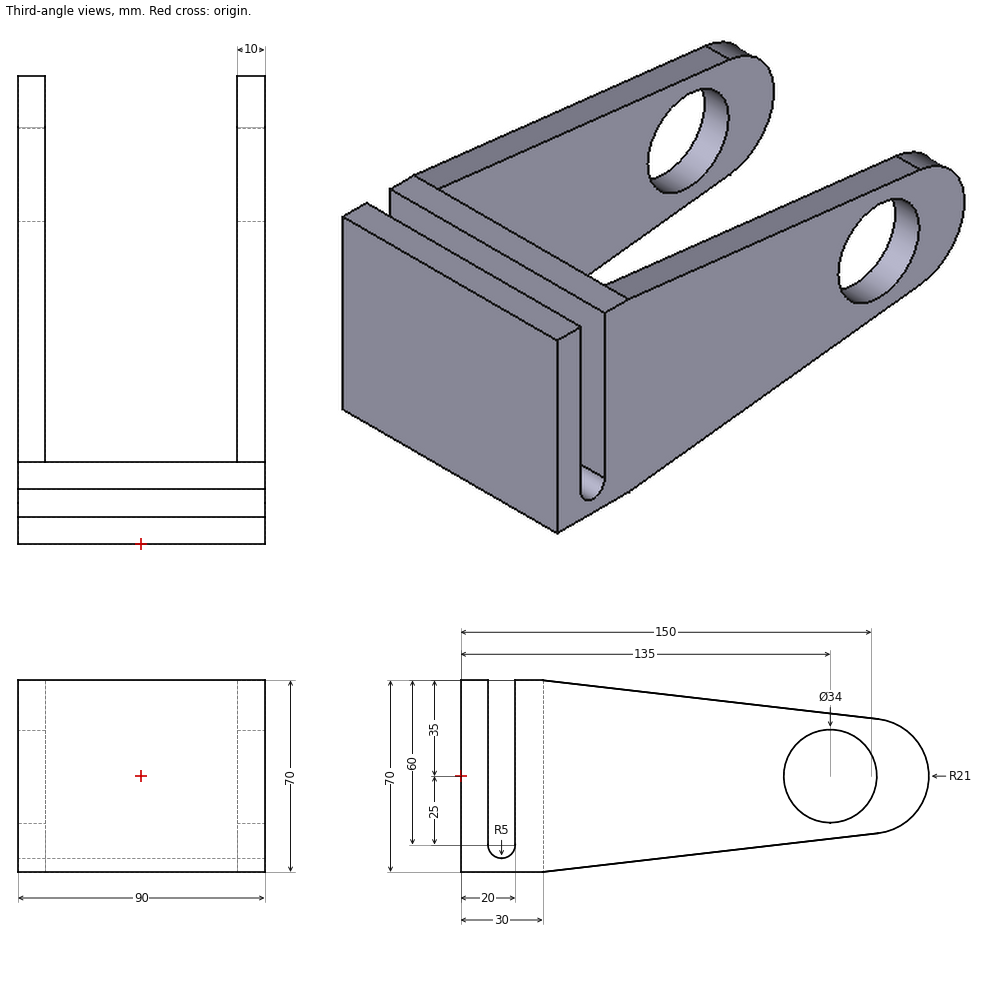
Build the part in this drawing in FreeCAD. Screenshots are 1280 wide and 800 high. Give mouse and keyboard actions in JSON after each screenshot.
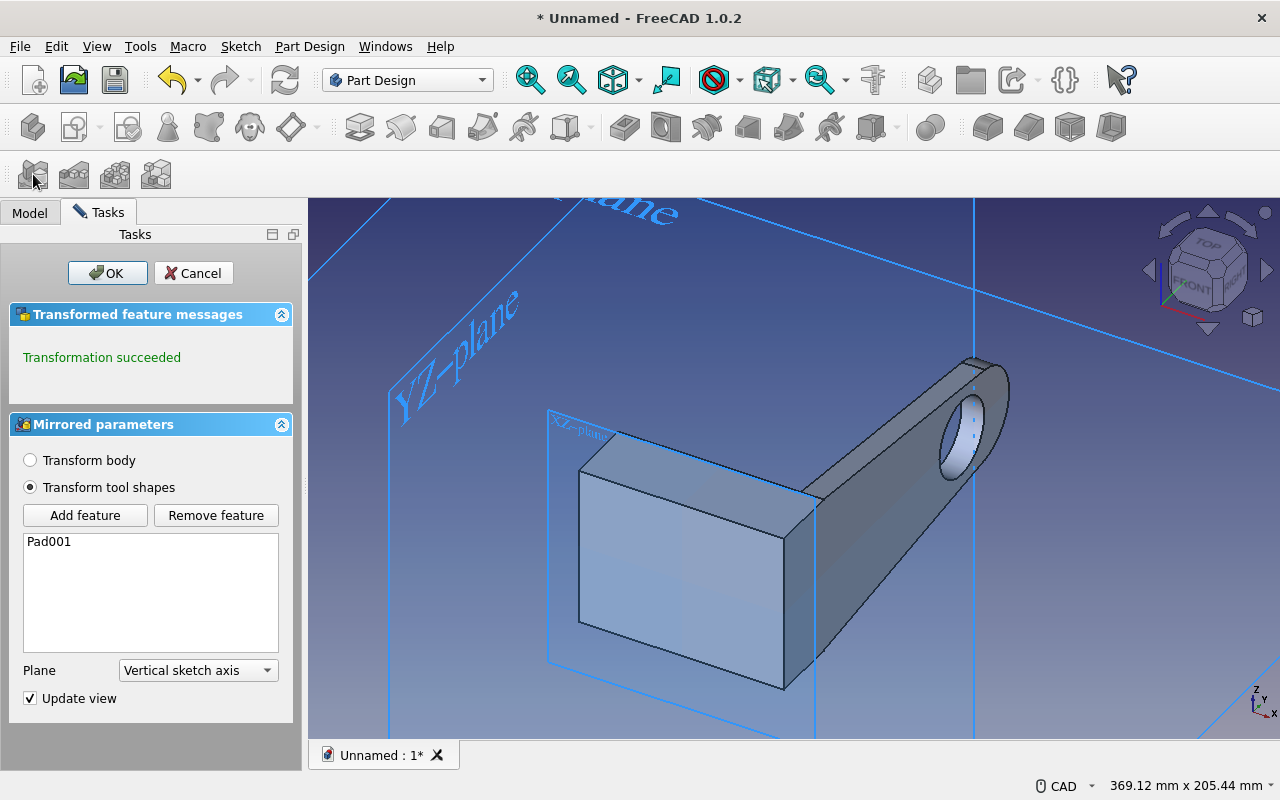
{"action": "left_click", "coordinate": [199, 670]}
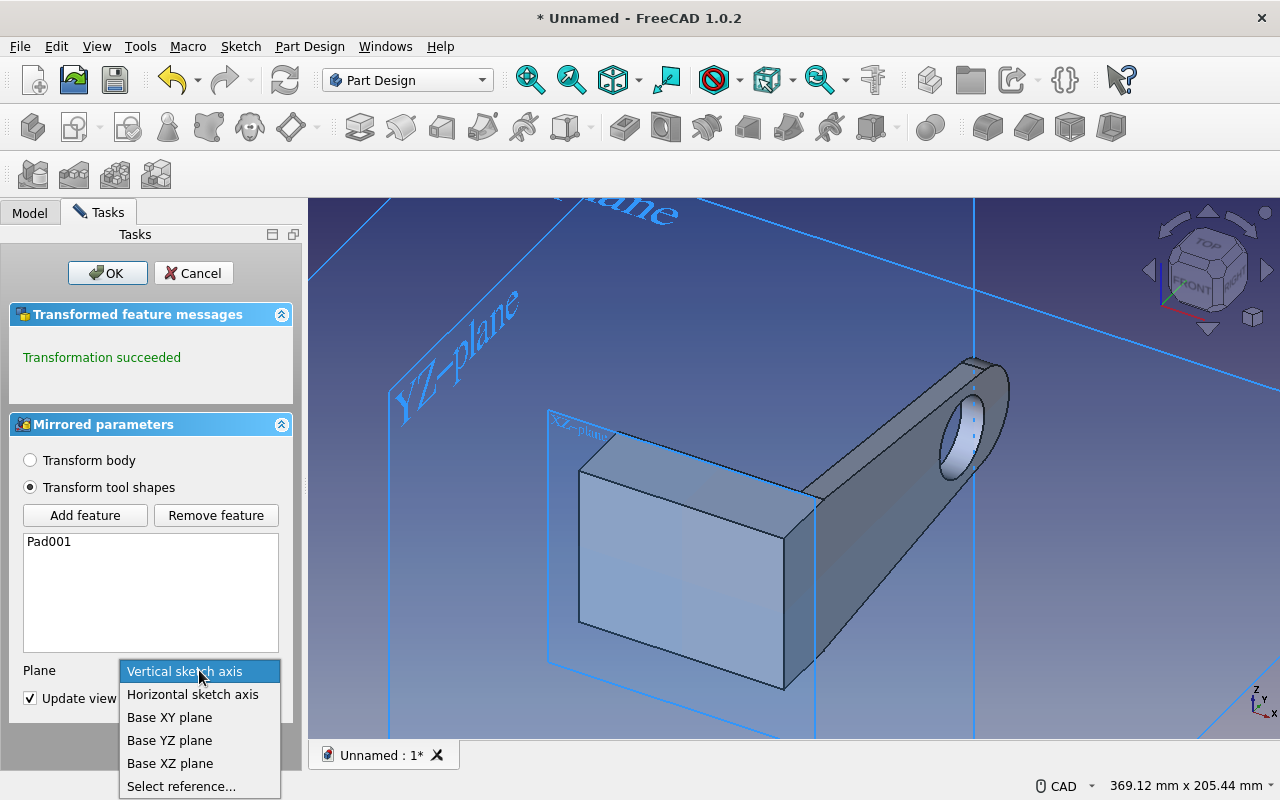
{"action": "left_click", "coordinate": [198, 740]}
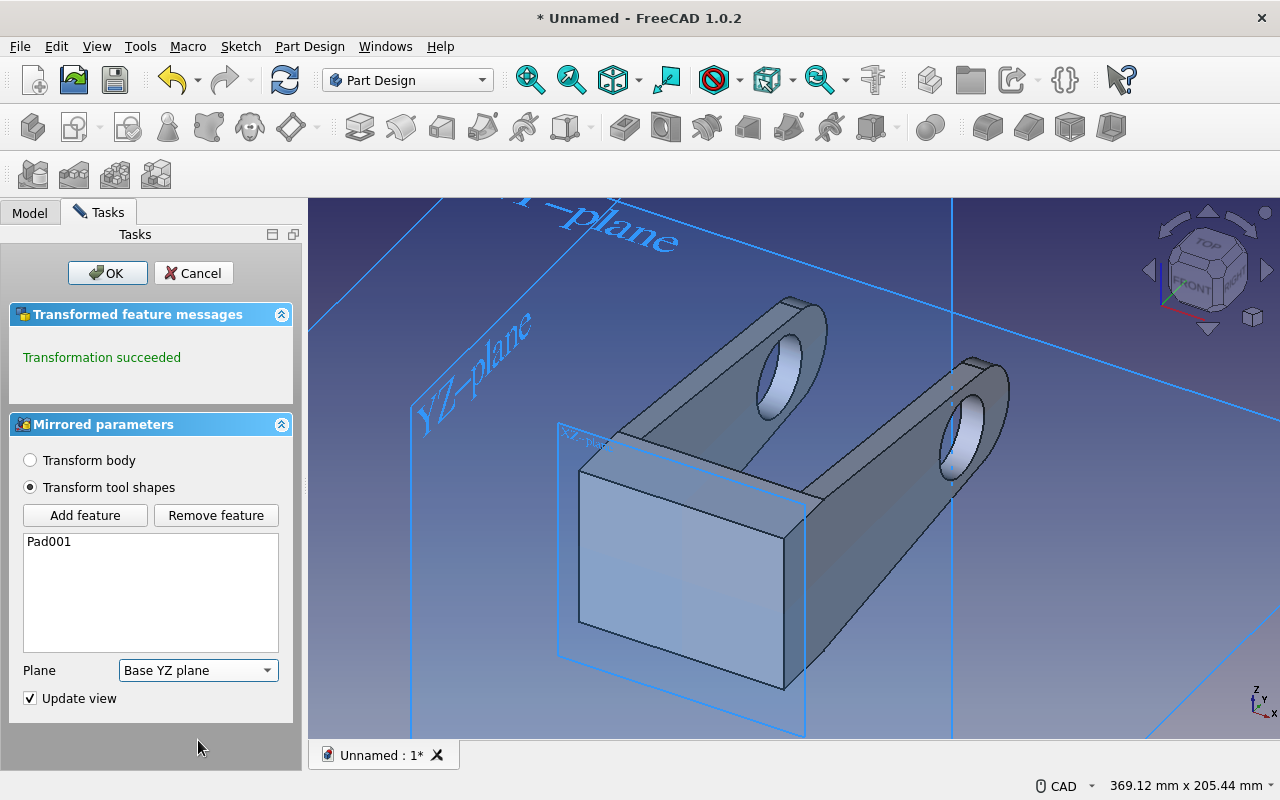
{"action": "left_click", "coordinate": [108, 273]}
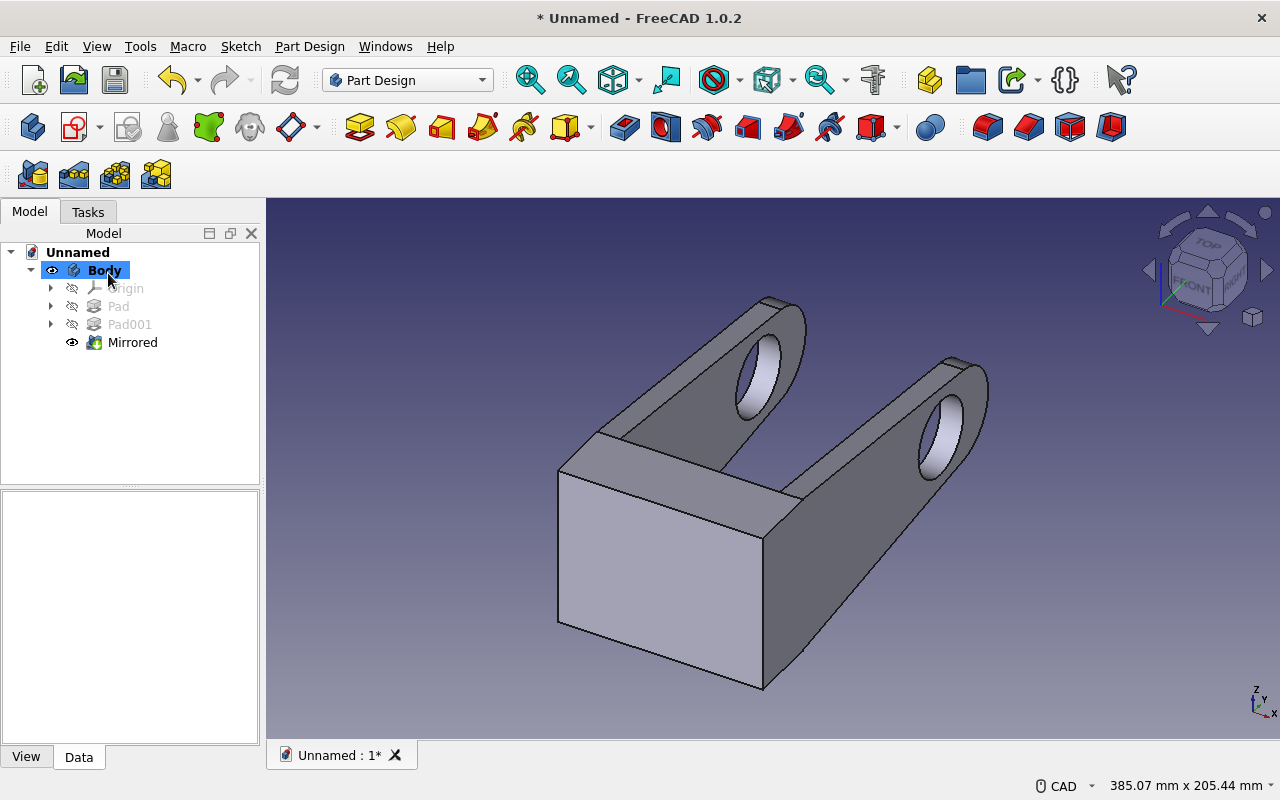
{"action": "left_click", "coordinate": [811, 565]}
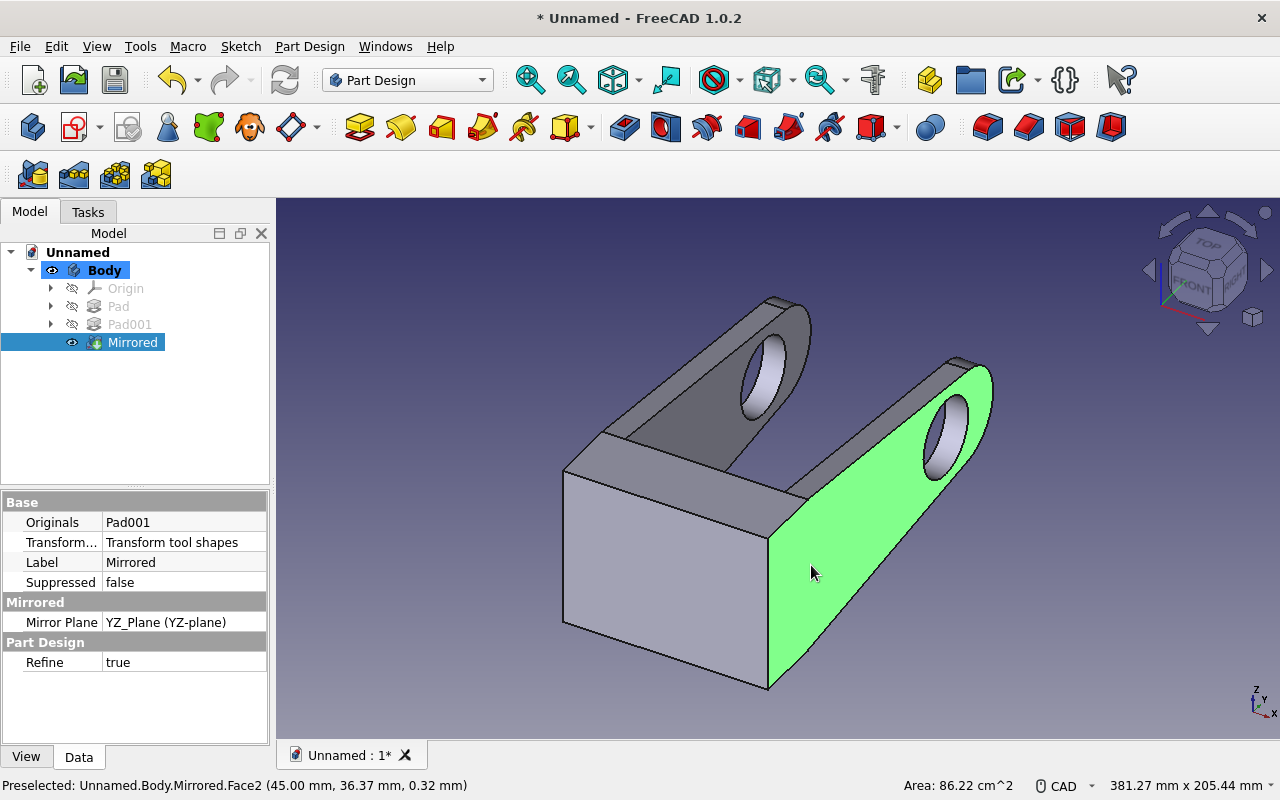
{"action": "left_click", "coordinate": [74, 128]}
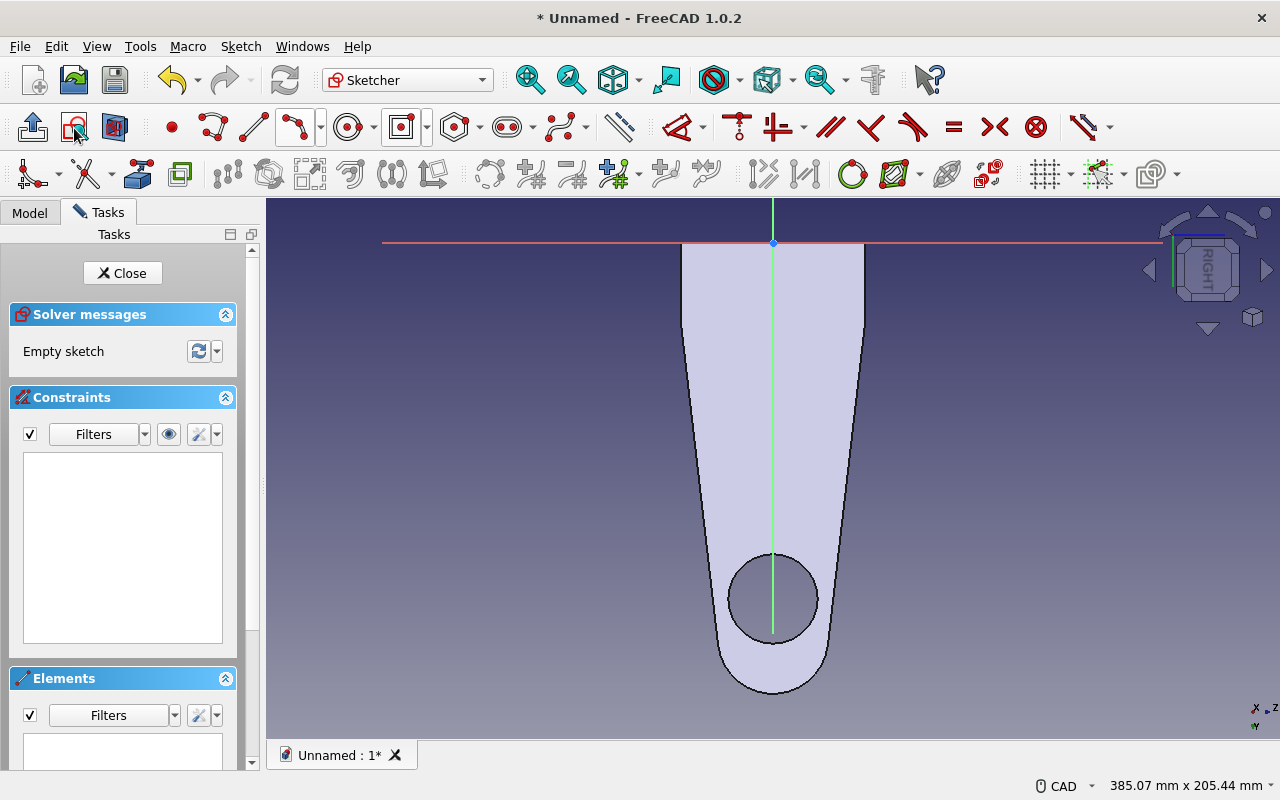
{"action": "scroll", "coordinate": [812, 226], "scroll_direction": "up", "scroll_amount": 6}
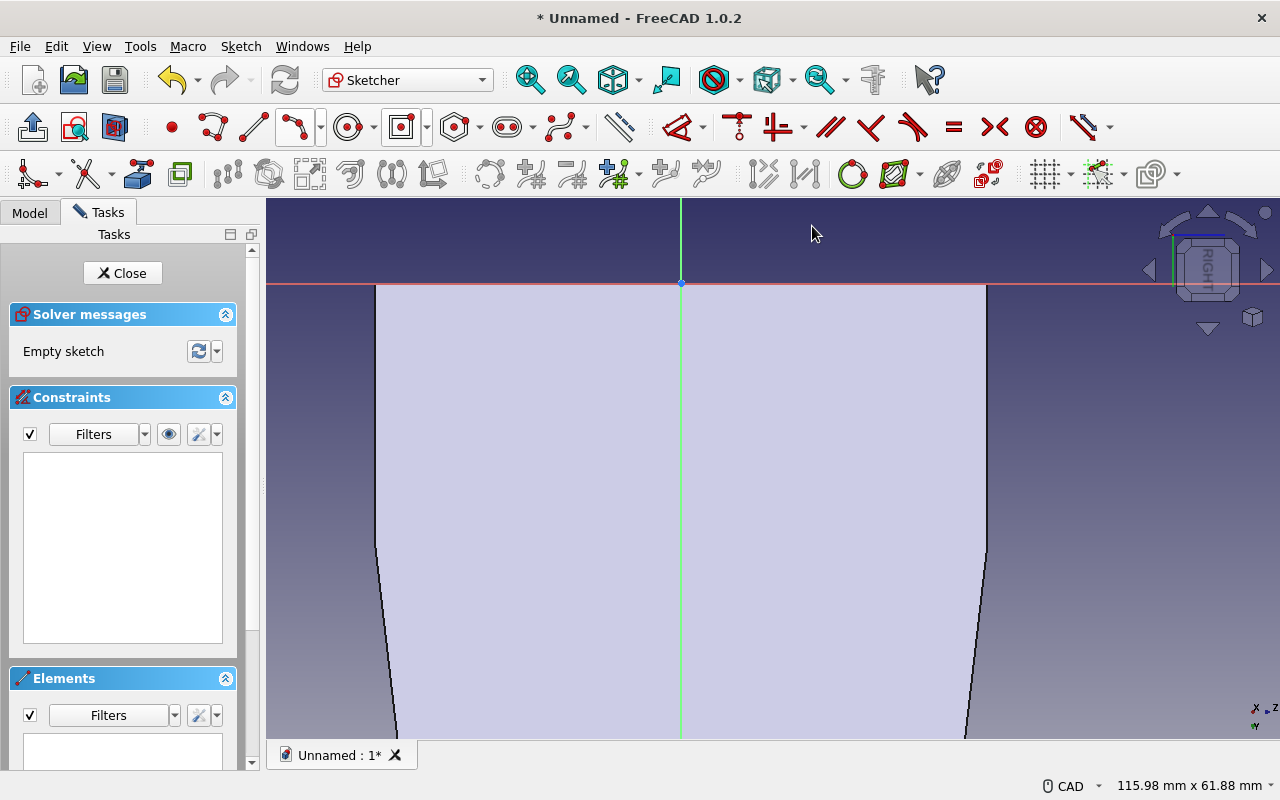
{"action": "left_click", "coordinate": [213, 128]}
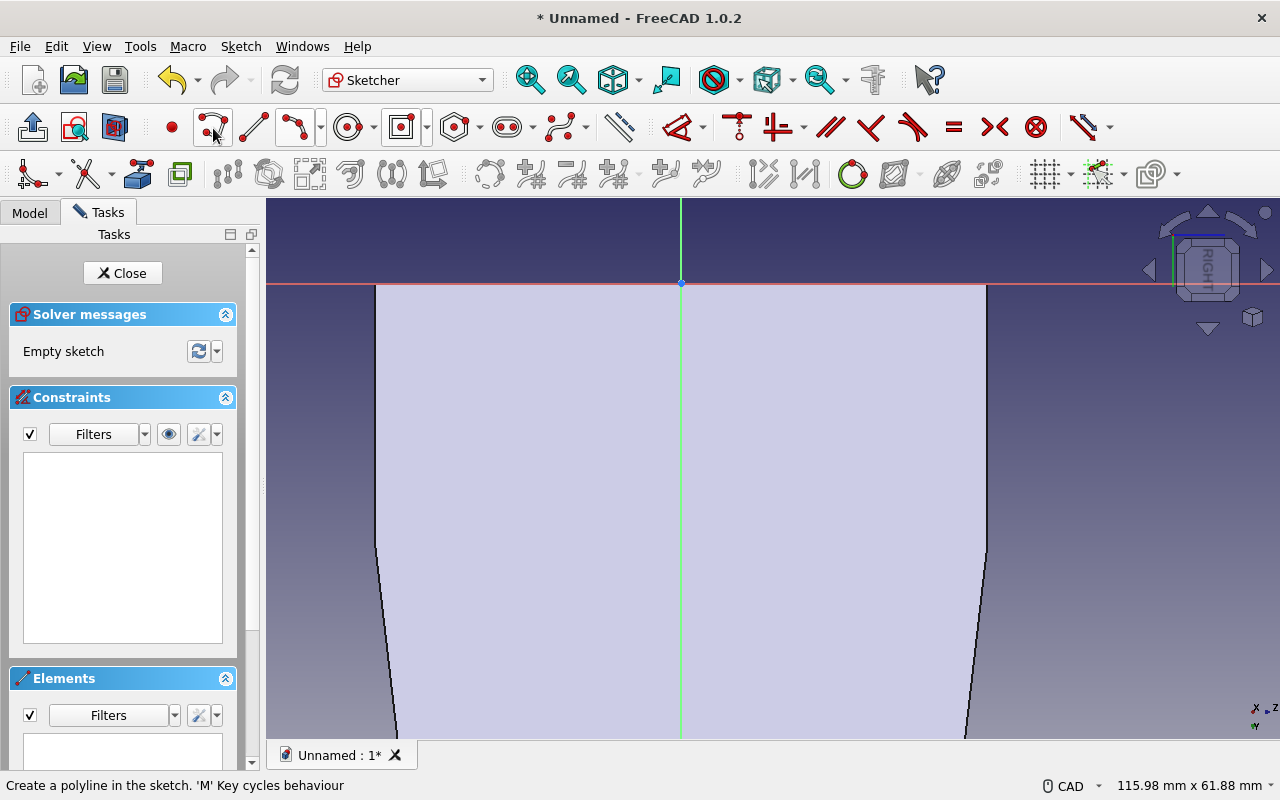
{"action": "left_click", "coordinate": [463, 459]}
{"action": "left_click", "coordinate": [987, 459]}
{"action": "left_click", "coordinate": [987, 371]}
{"action": "left_click", "coordinate": [463, 371]}
{"action": "right_click", "coordinate": [463, 371]}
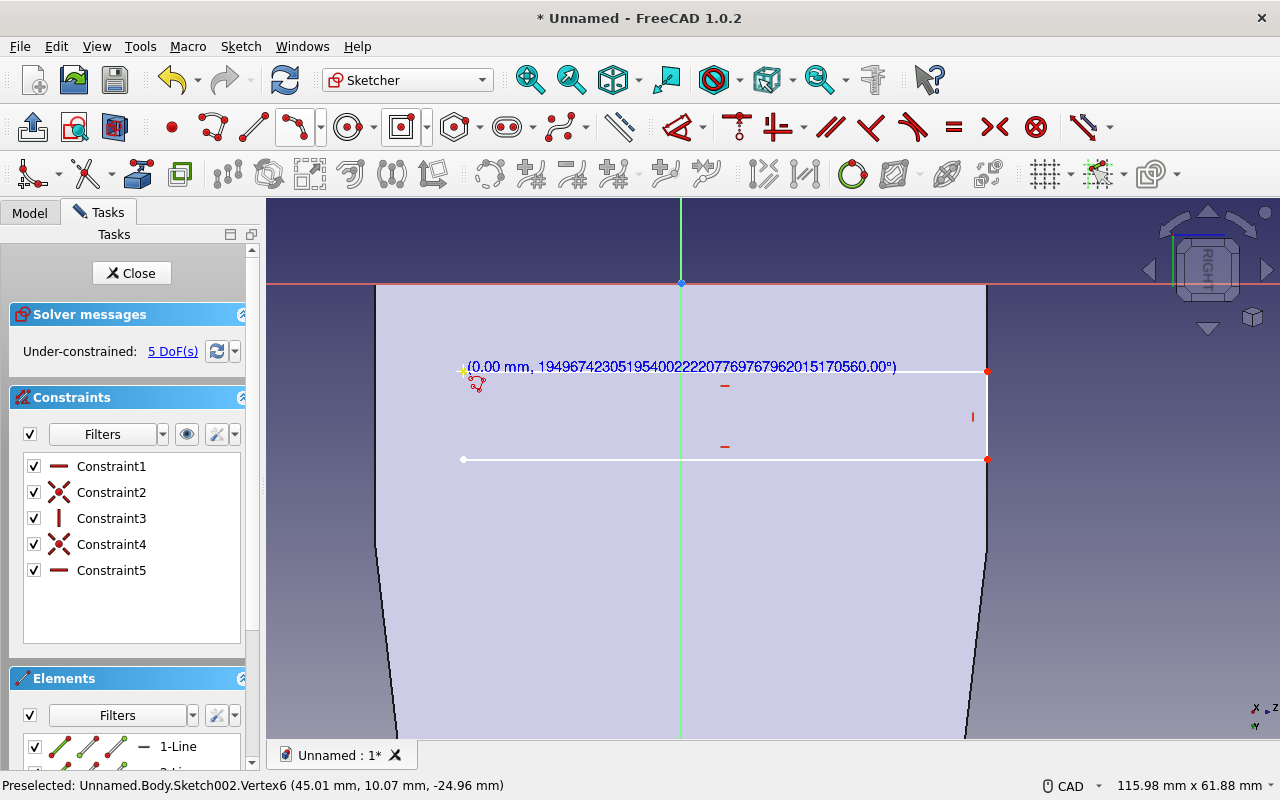
{"action": "left_click", "coordinate": [294, 128]}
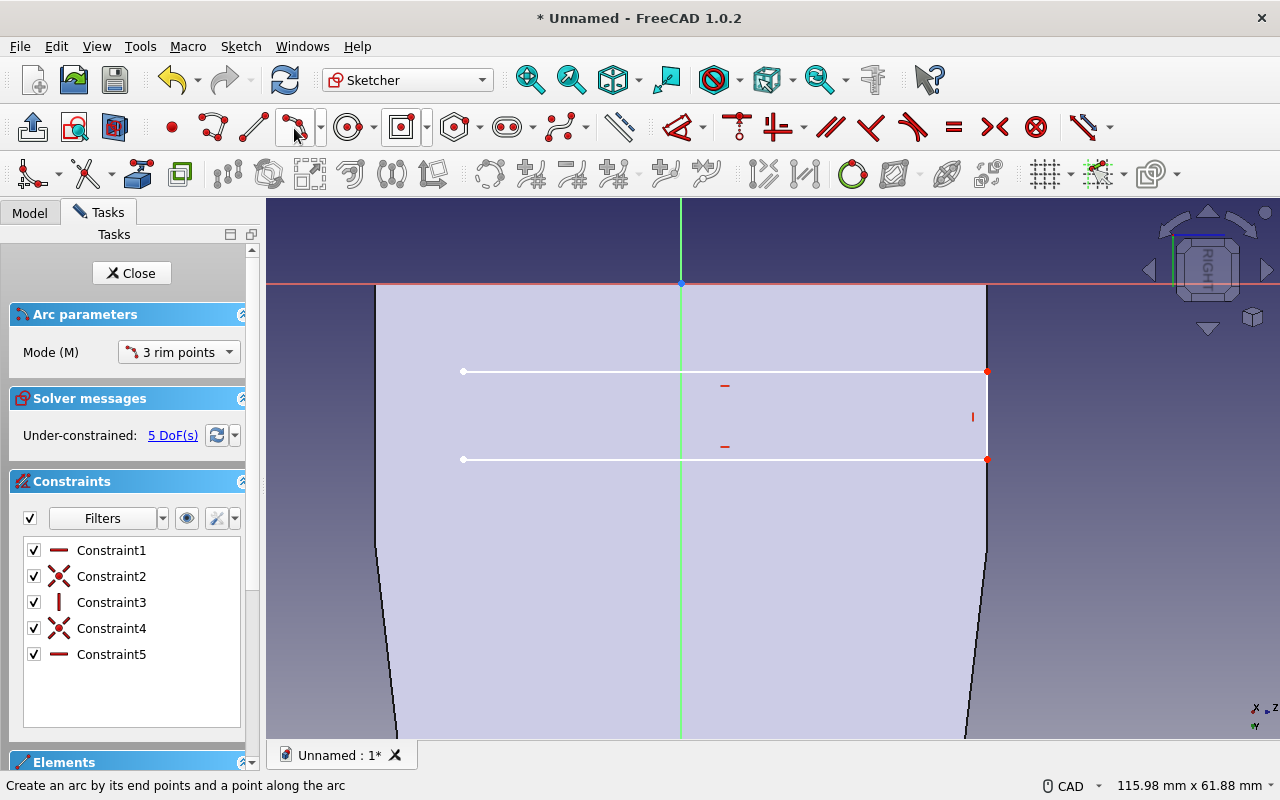
{"action": "left_click", "coordinate": [463, 372]}
{"action": "left_click", "coordinate": [463, 460]}
{"action": "left_click", "coordinate": [419, 415]}
{"action": "key", "text": "Escape"}